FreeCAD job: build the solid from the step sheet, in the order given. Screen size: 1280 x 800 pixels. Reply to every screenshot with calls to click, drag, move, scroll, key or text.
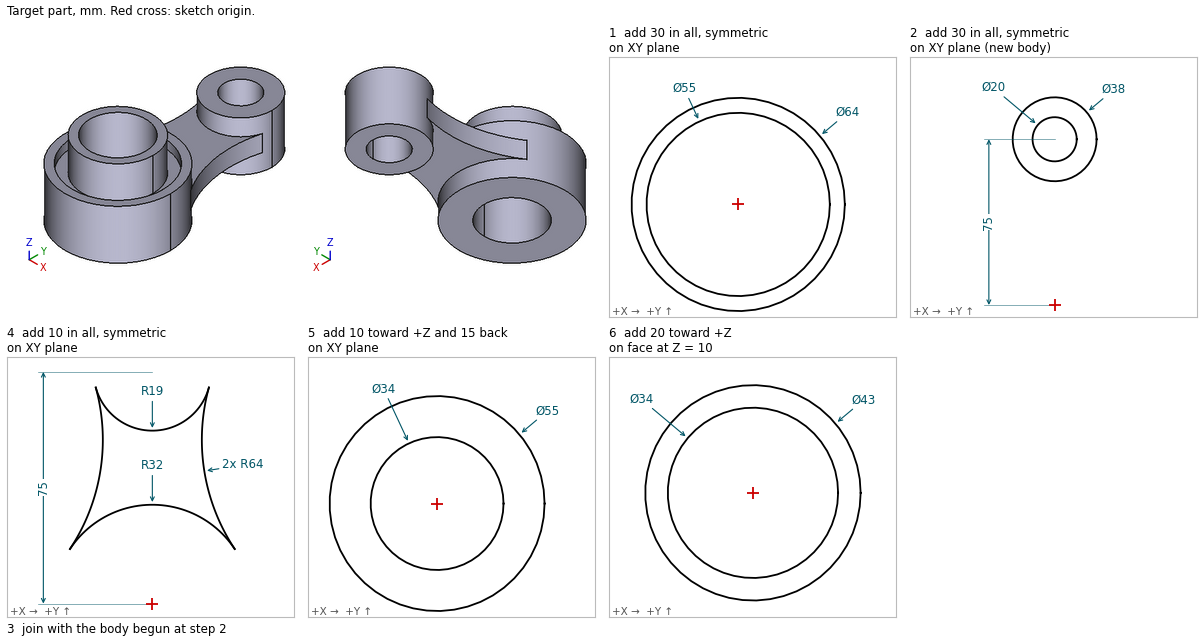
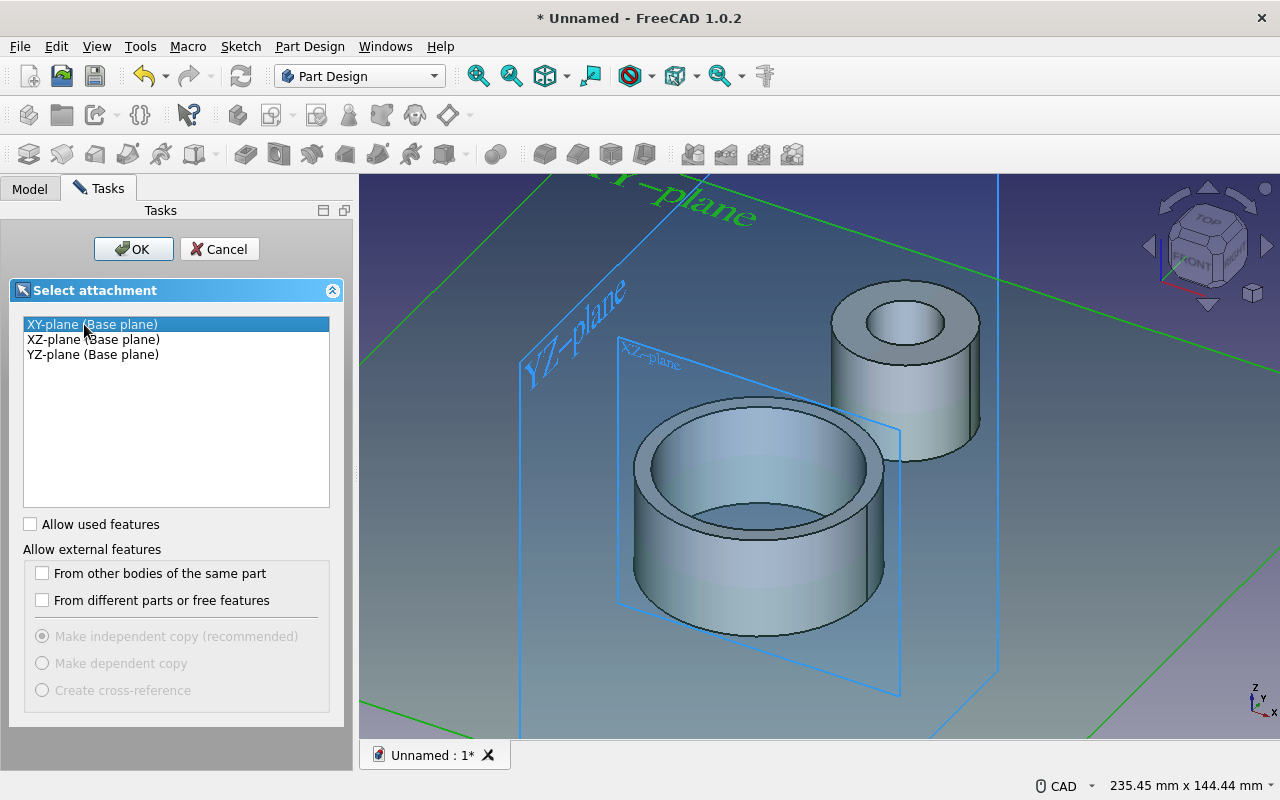
click(134, 249)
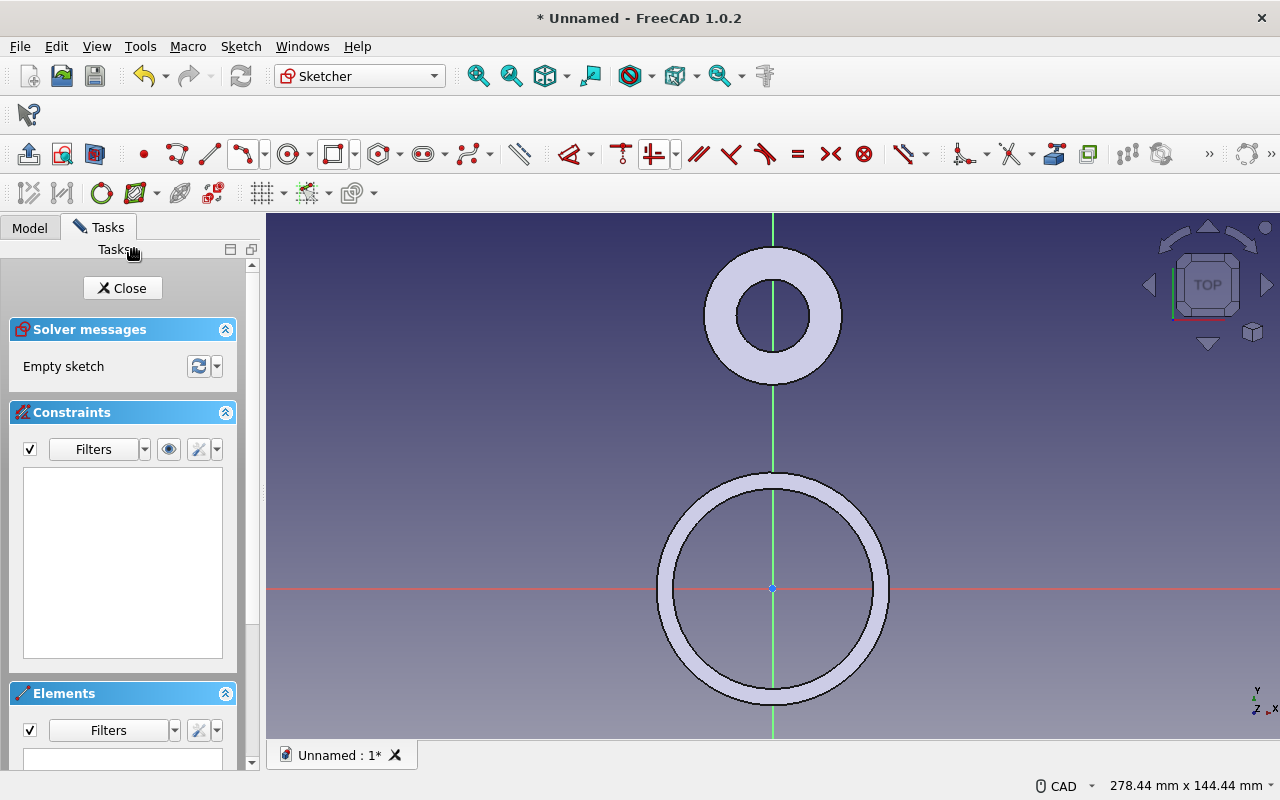
key(q)
key(s)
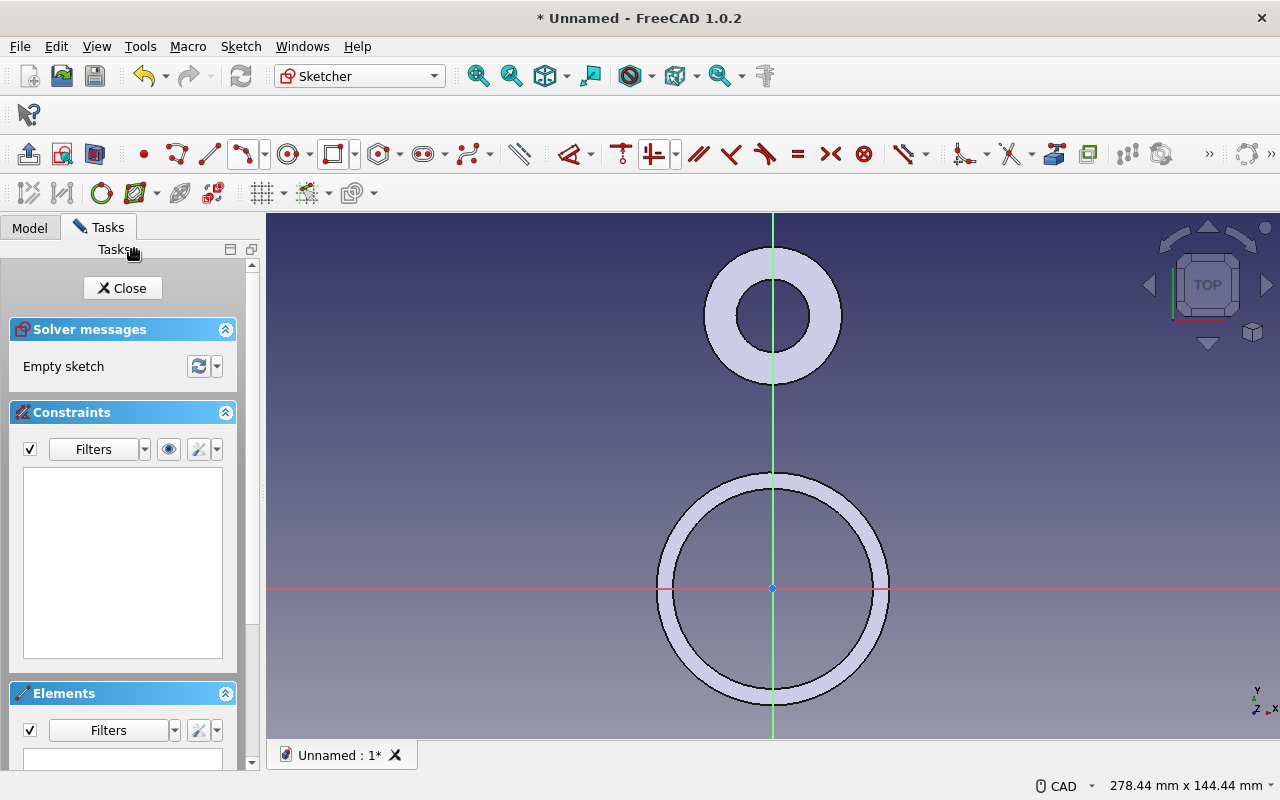
key(g)
key(3)
key(a)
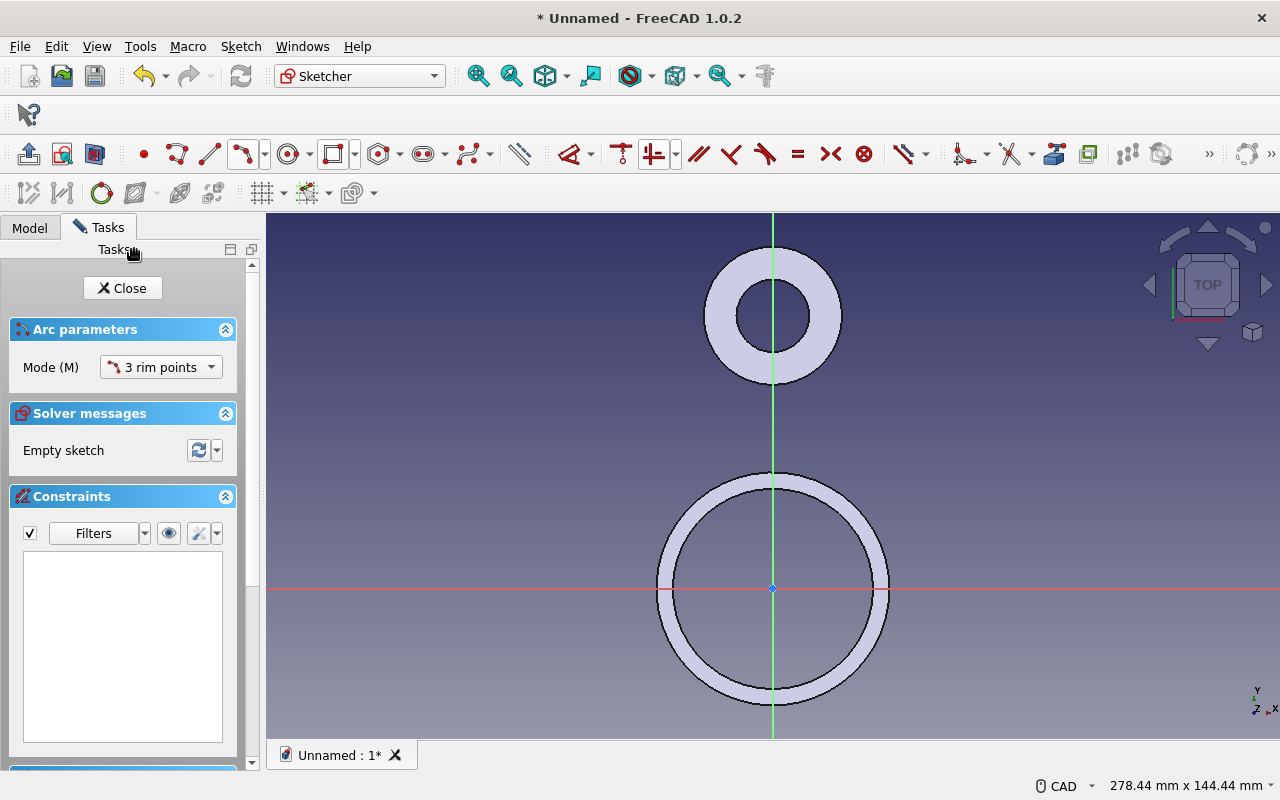
click(676, 525)
click(870, 525)
click(796, 475)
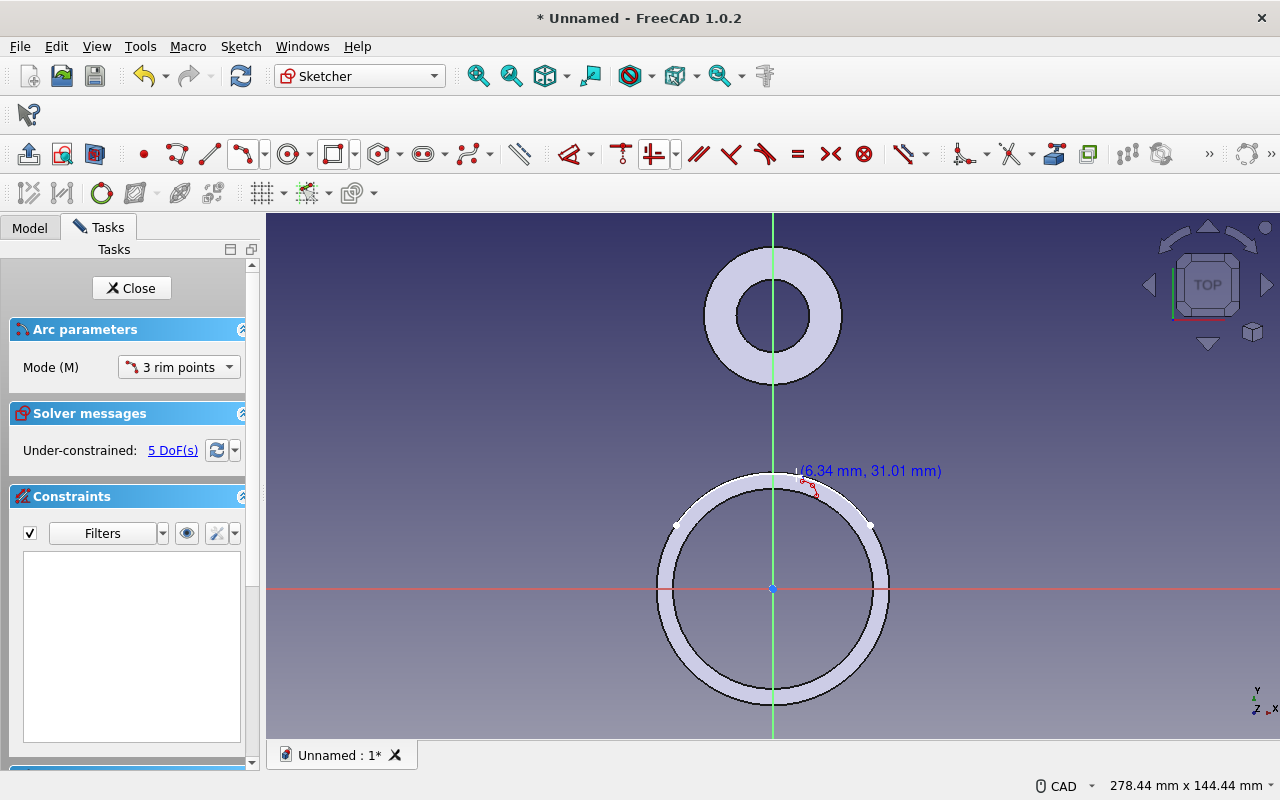
click(870, 526)
click(840, 334)
click(834, 433)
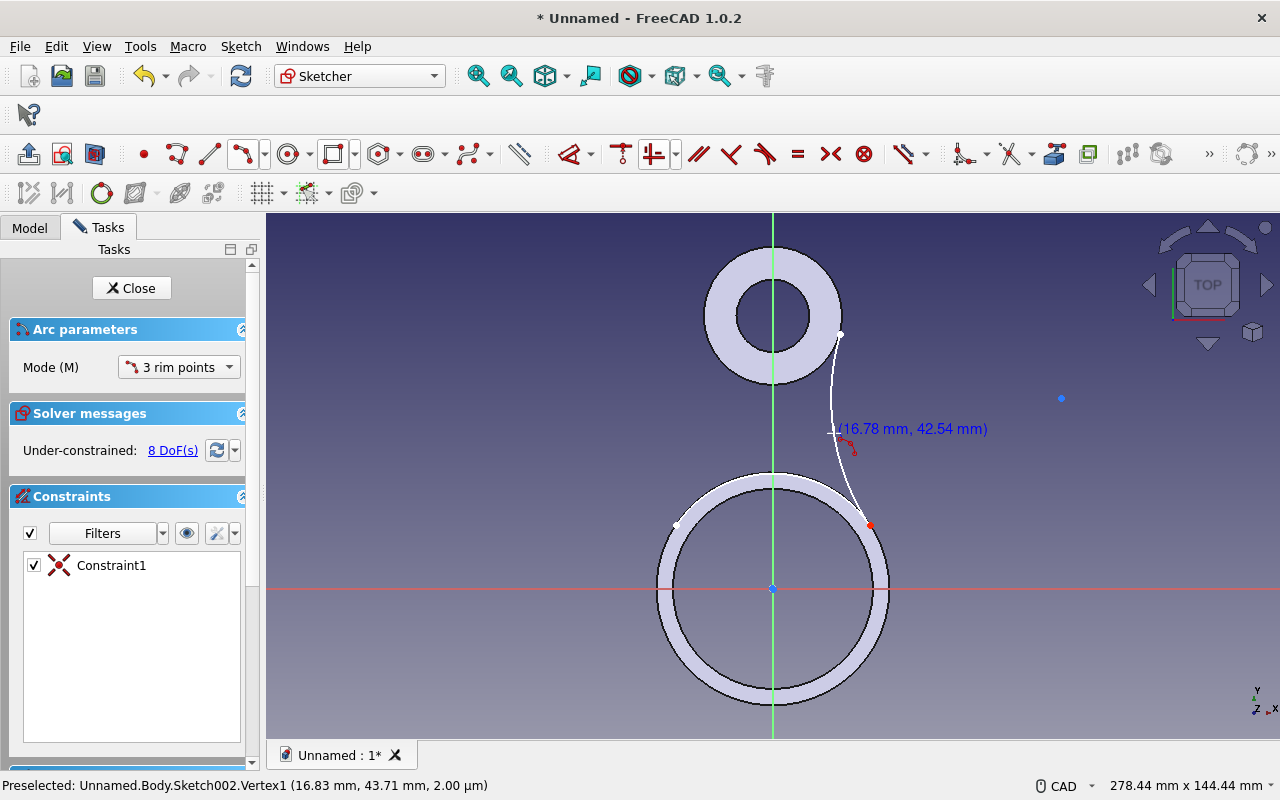
click(840, 335)
click(706, 334)
click(755, 383)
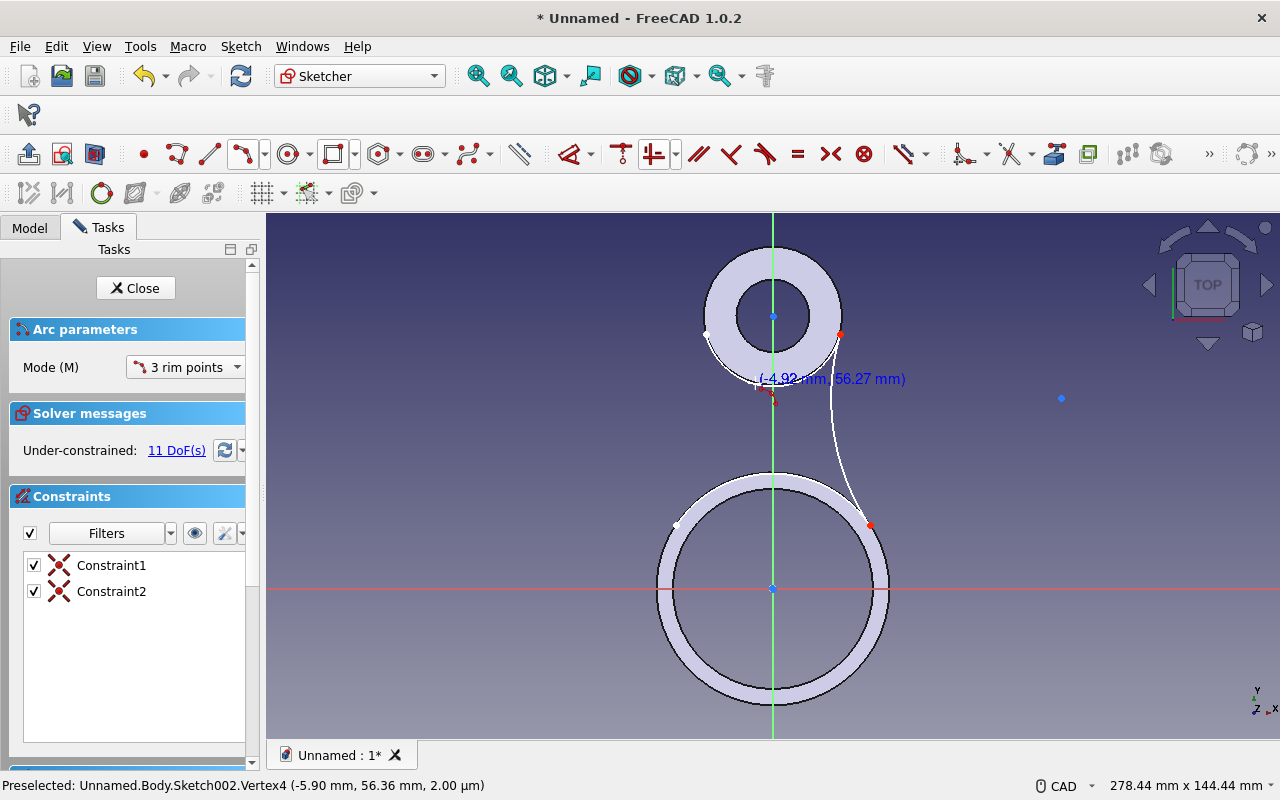
click(706, 335)
click(676, 526)
click(712, 433)
key(Escape)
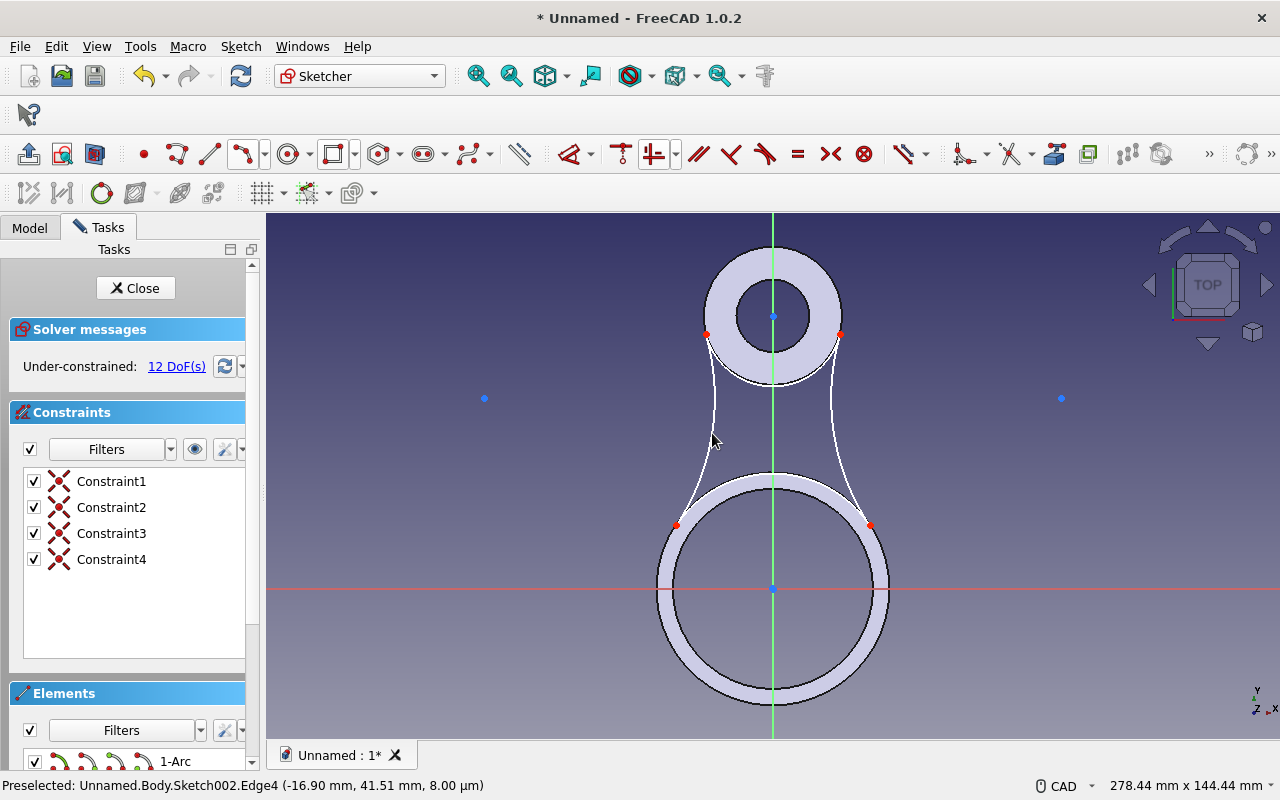
click(818, 483)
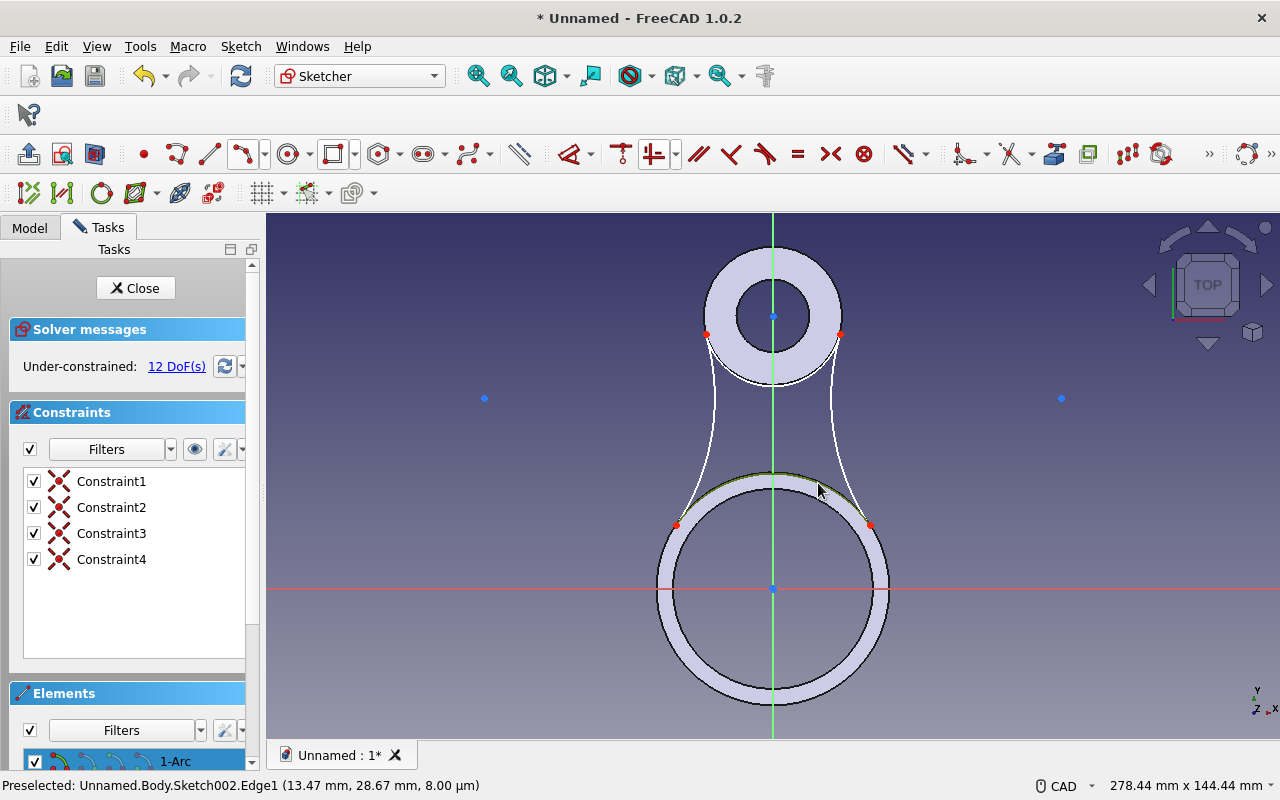
click(831, 394)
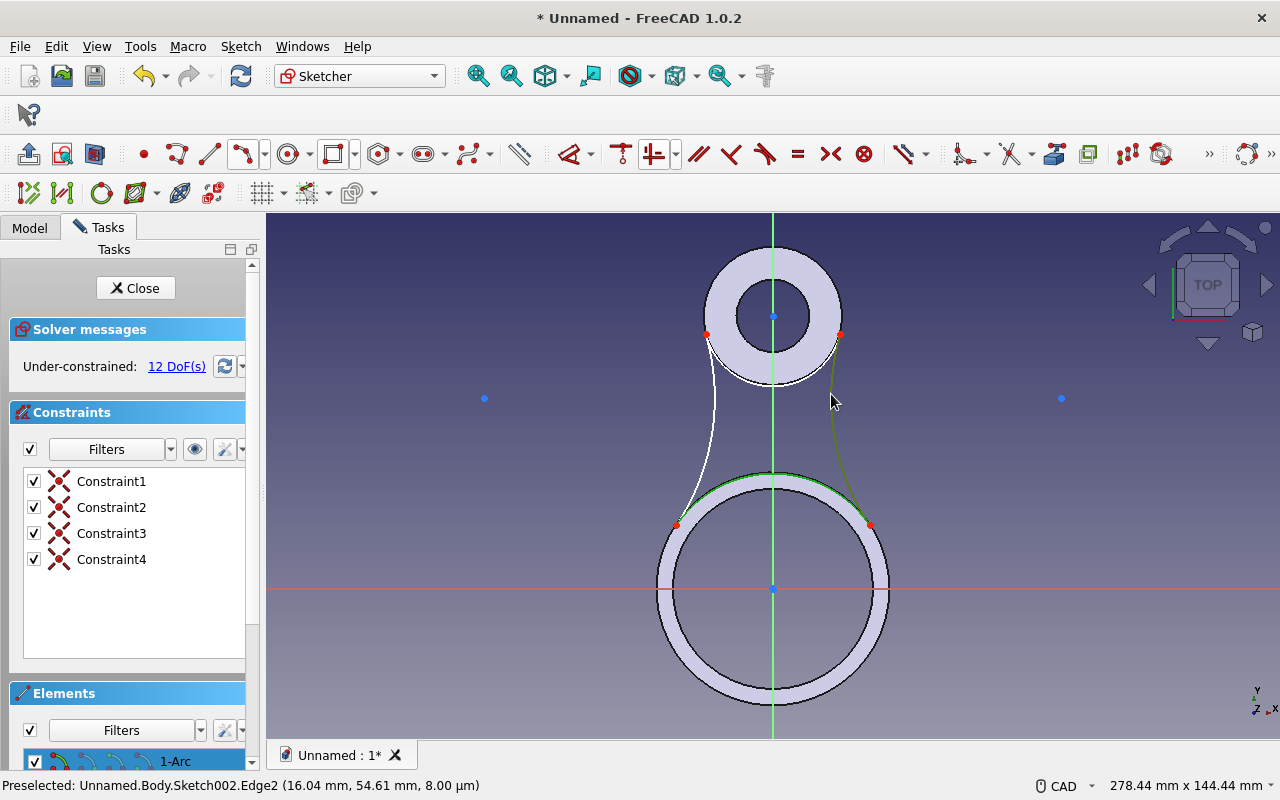
key(t)